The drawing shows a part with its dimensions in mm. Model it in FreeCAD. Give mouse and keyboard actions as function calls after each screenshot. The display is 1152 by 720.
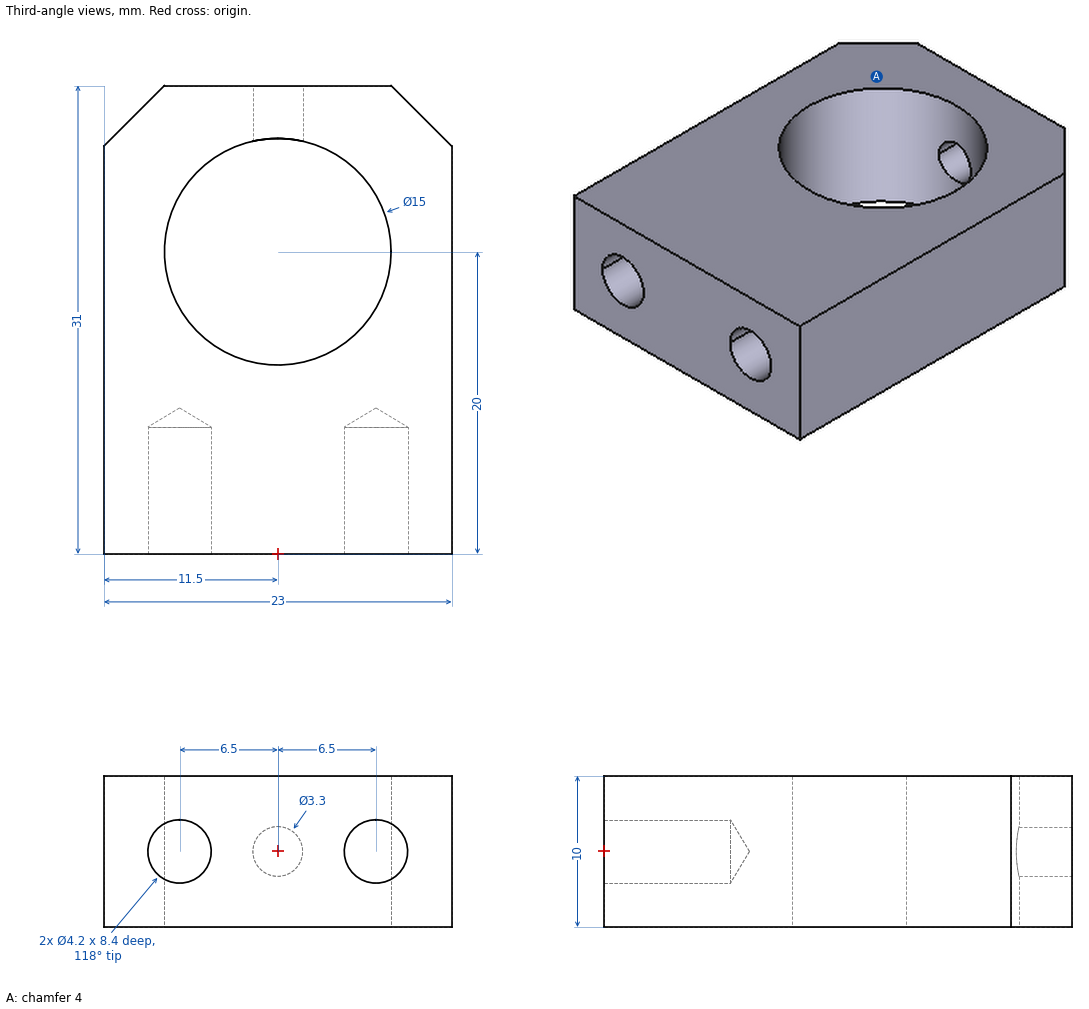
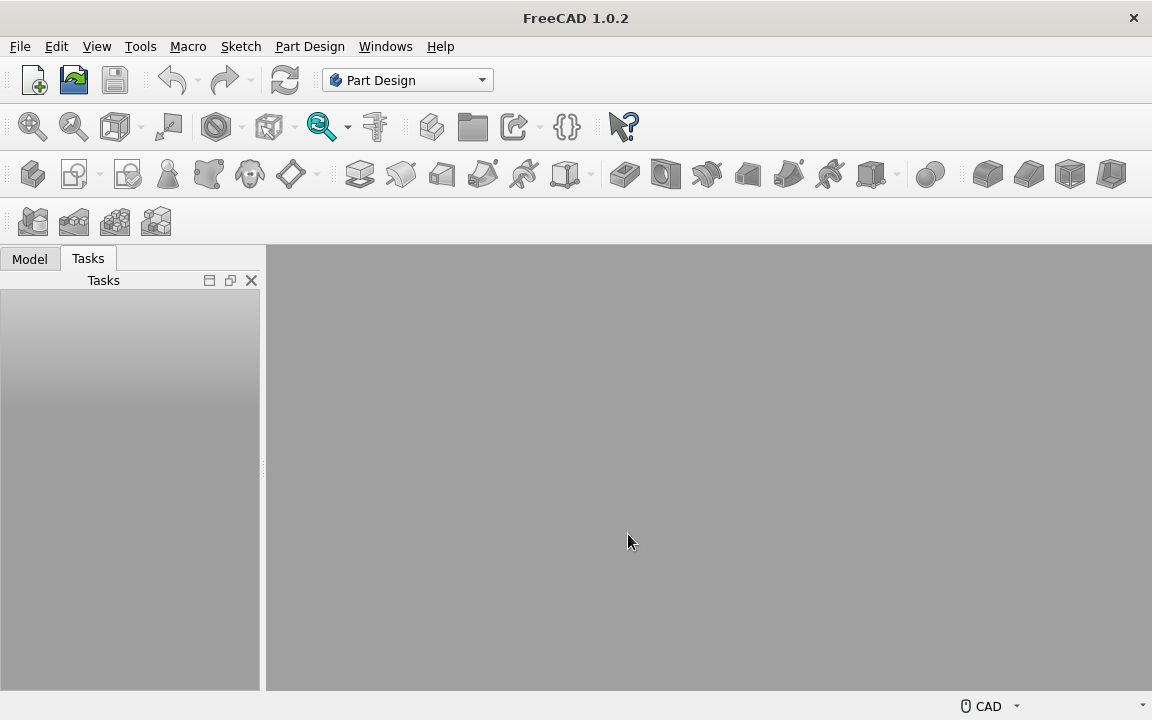
key(ctrl+n)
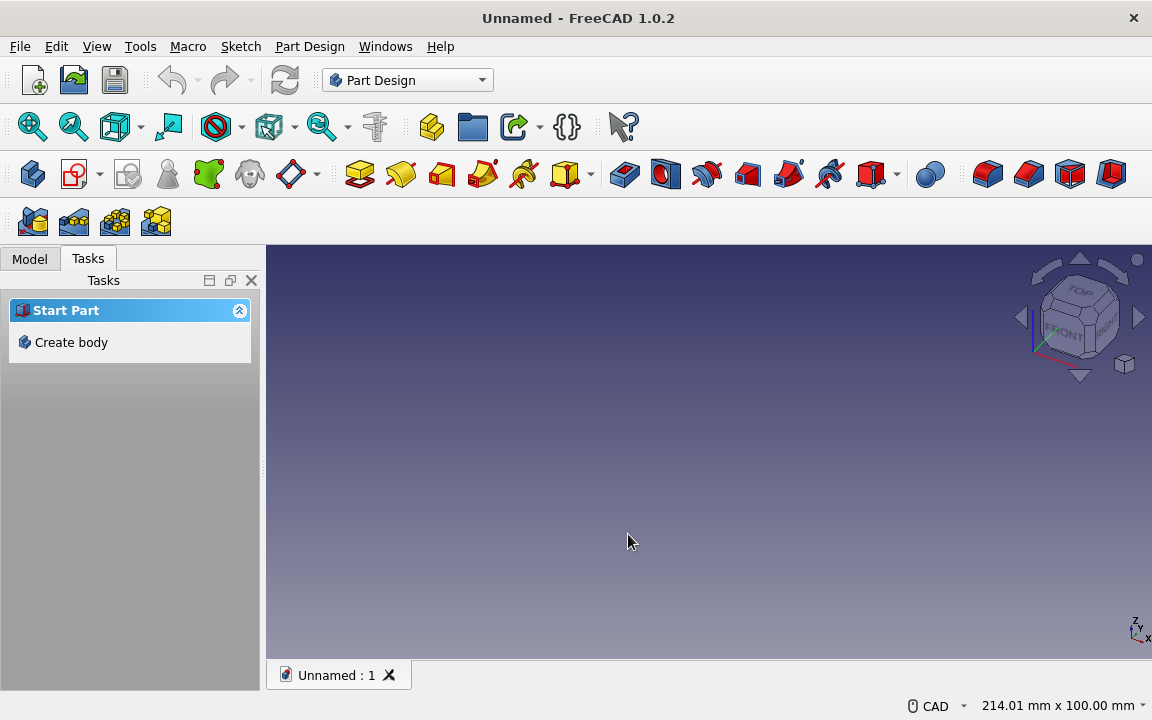
click(74, 174)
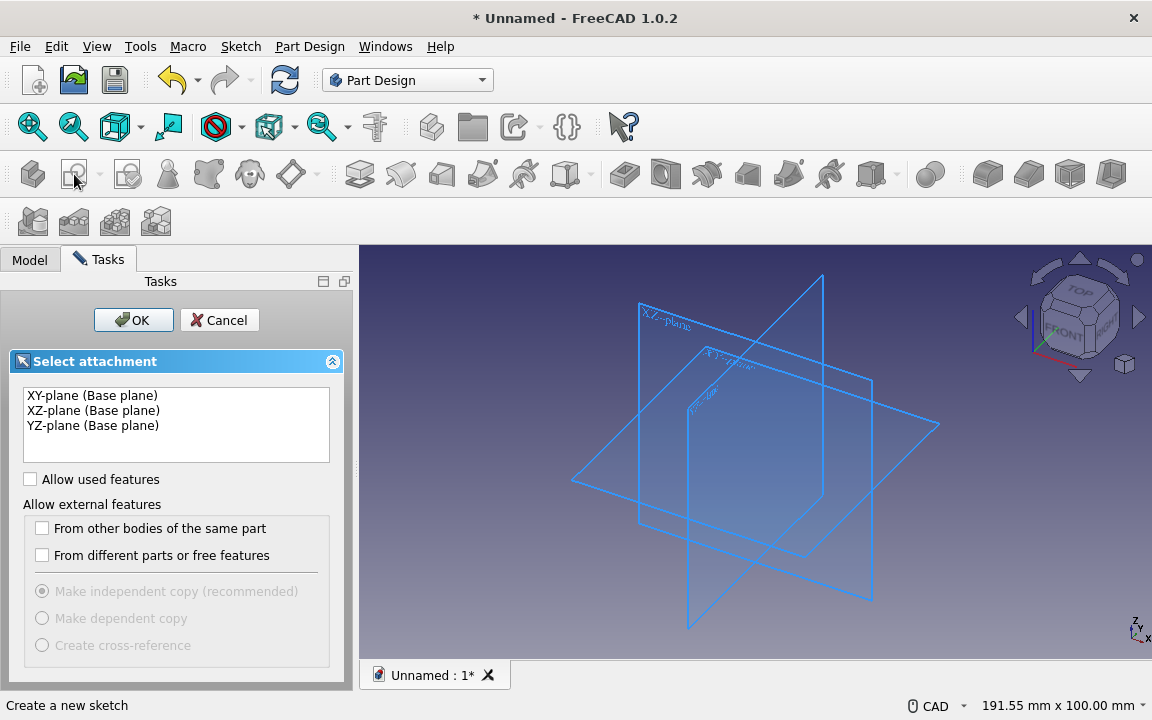
click(84, 396)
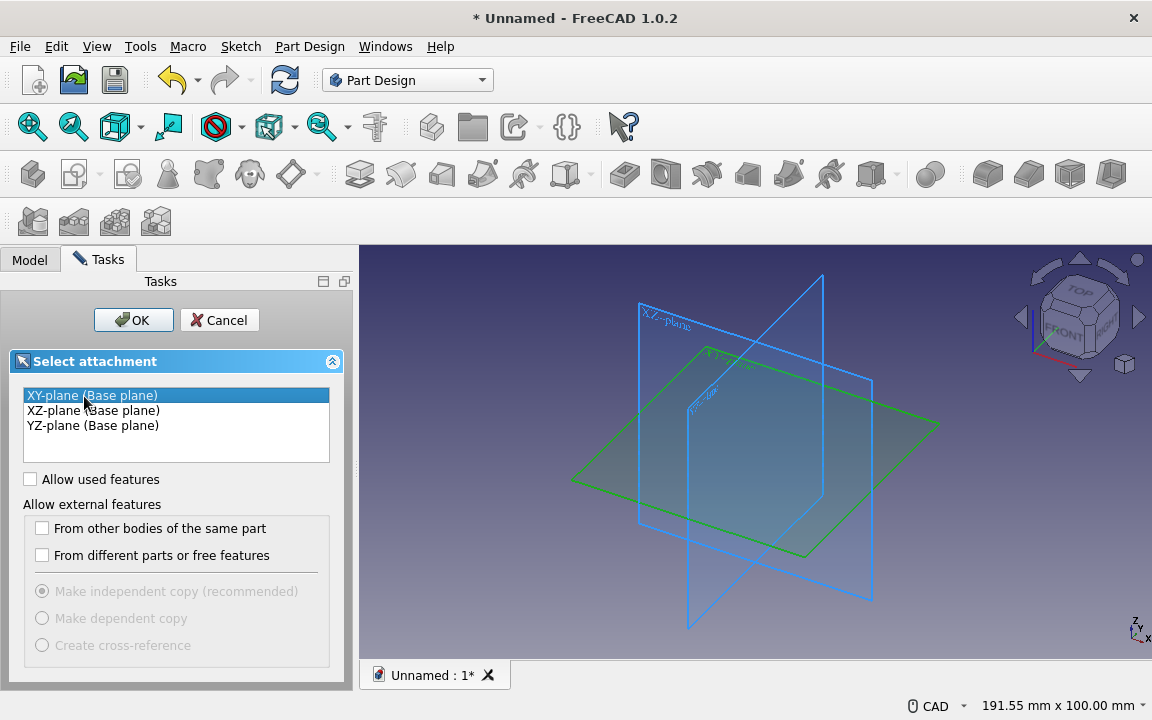
click(134, 320)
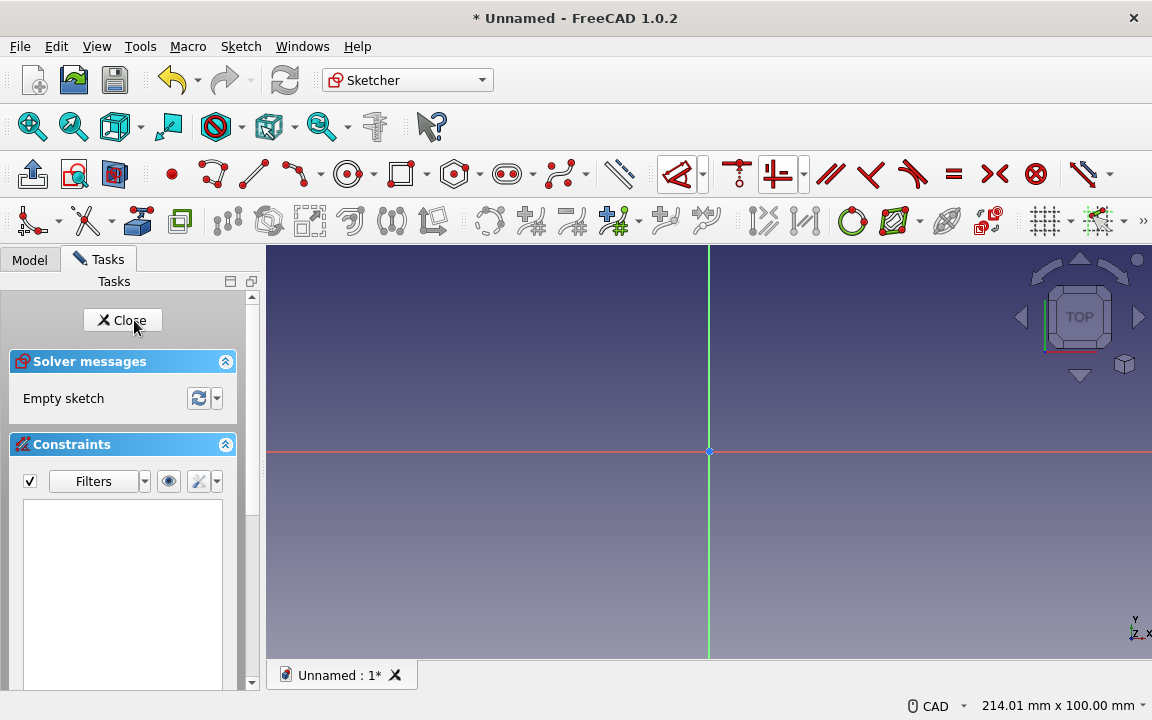
scroll(792, 310, up, 3)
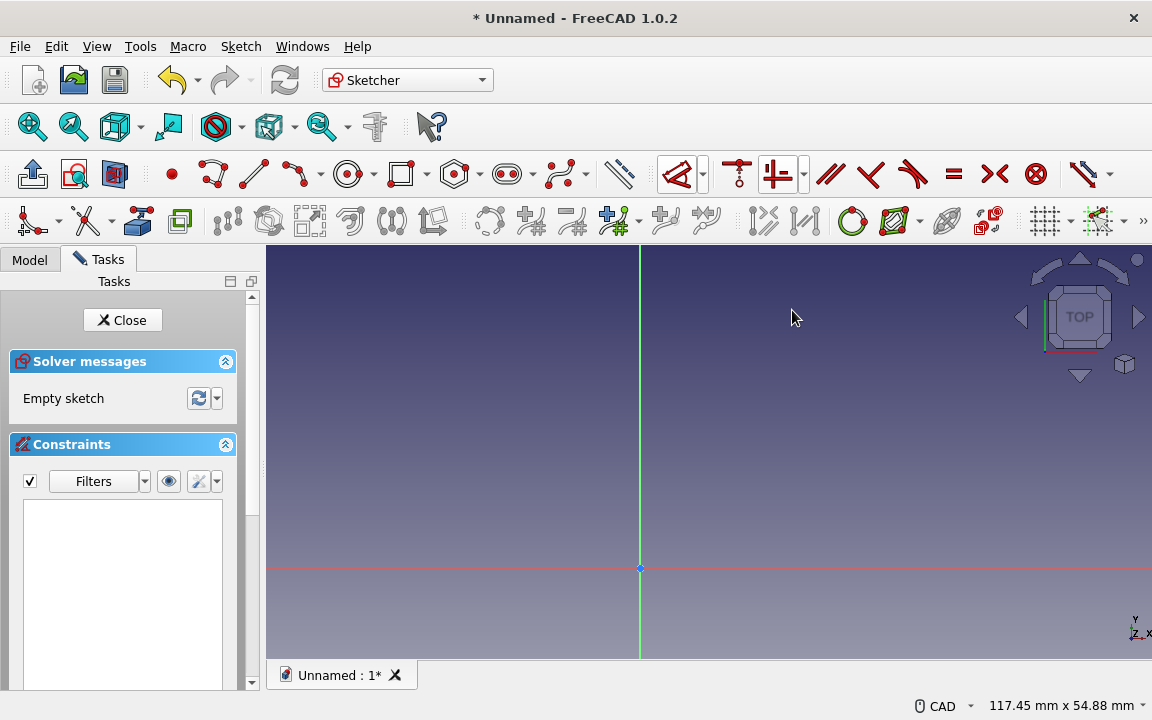
key(g)
key(r)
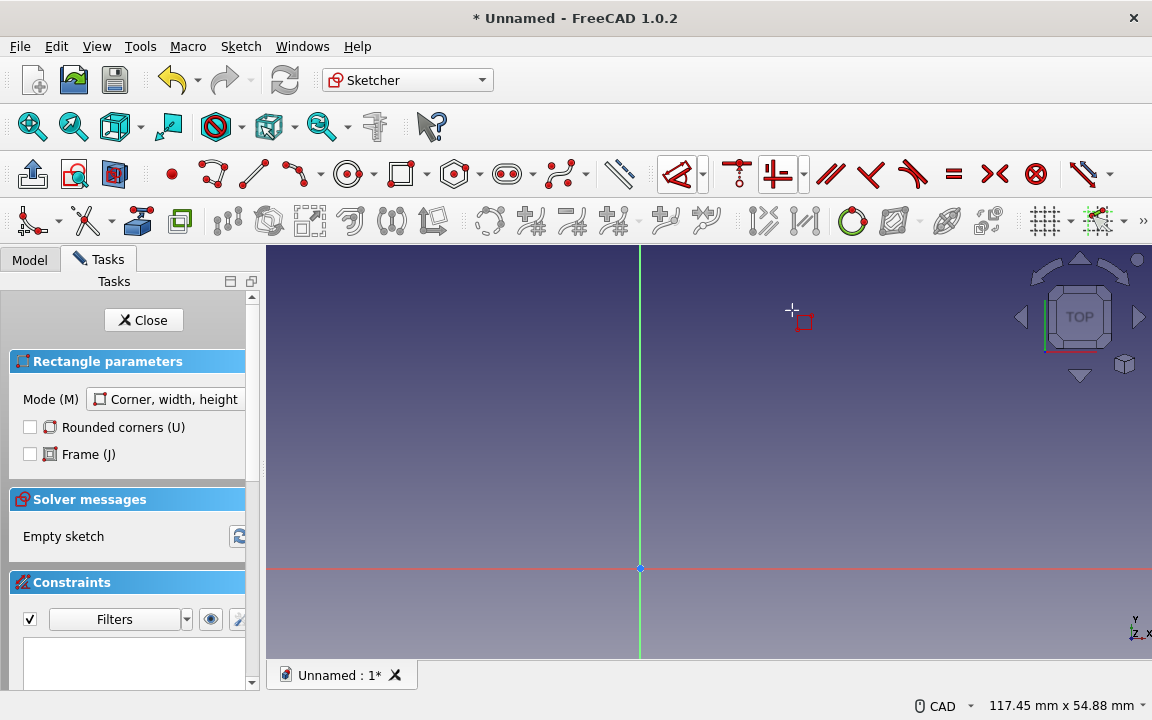
click(554, 335)
click(727, 569)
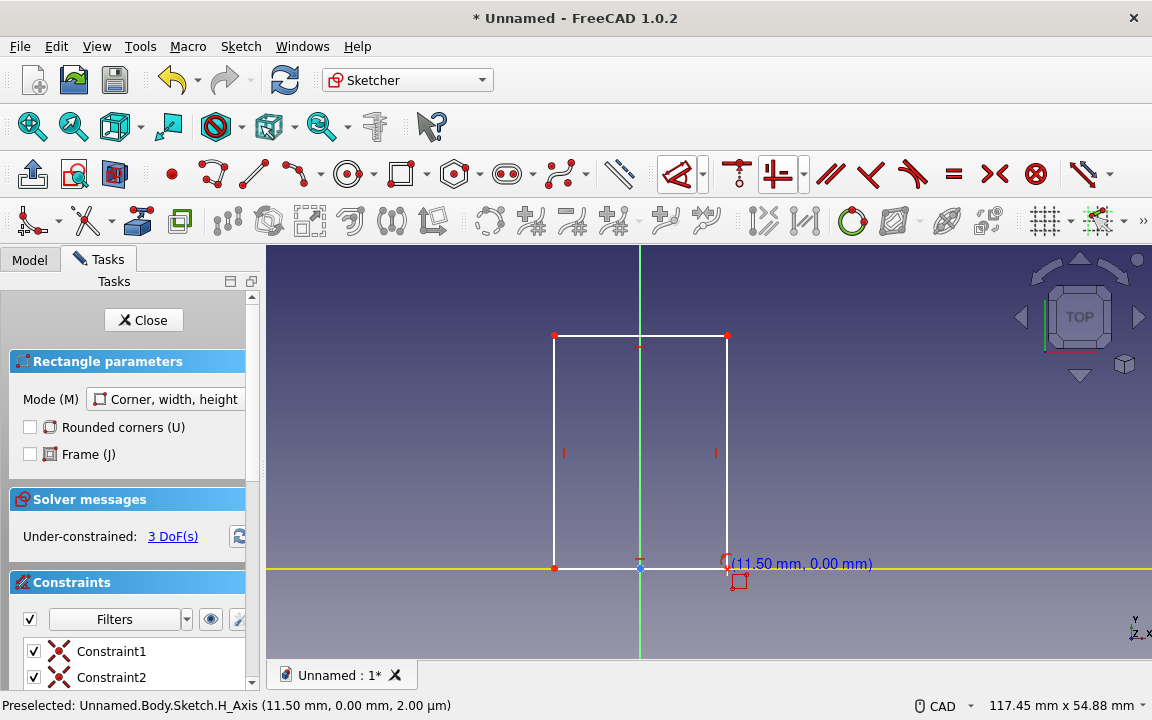
key(g)
key(c)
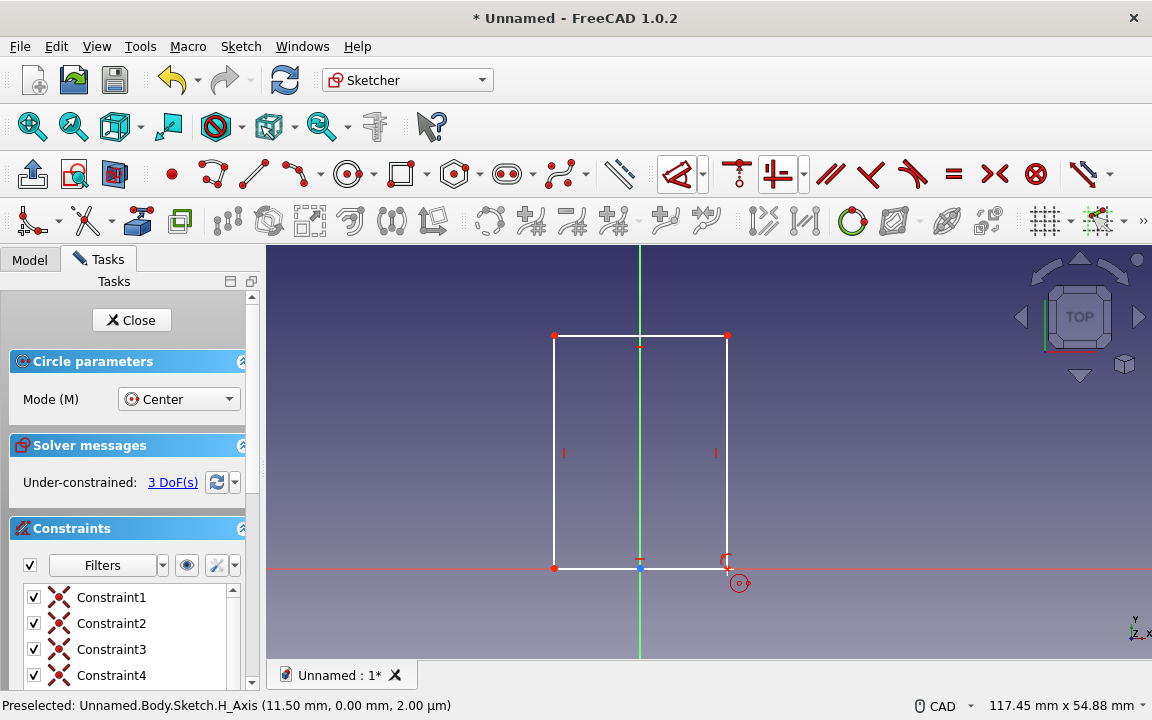
click(640, 418)
move(680, 378)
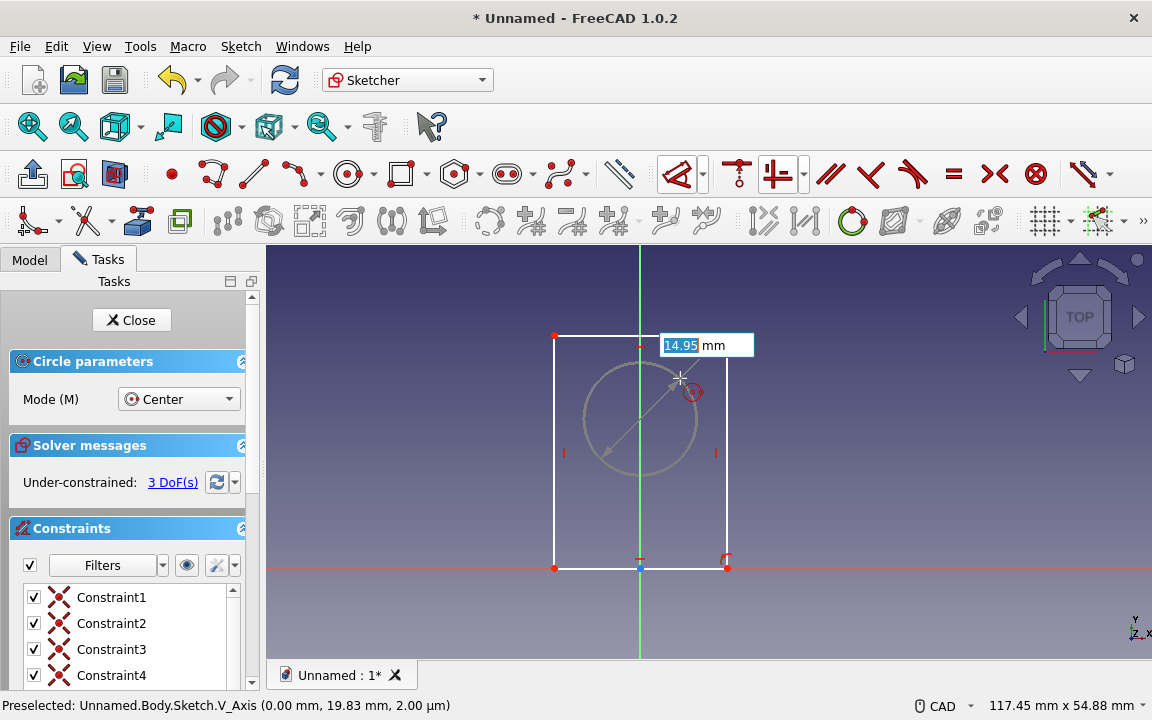
text(15)
key(Return)
key(Escape)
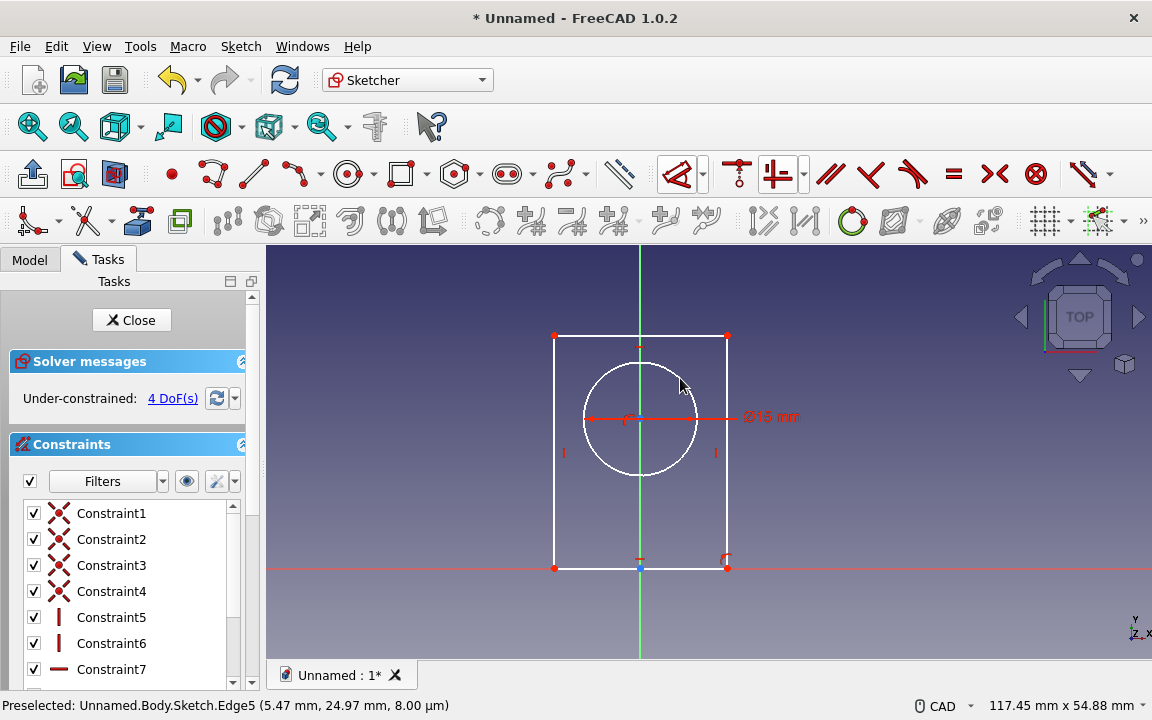
key(d)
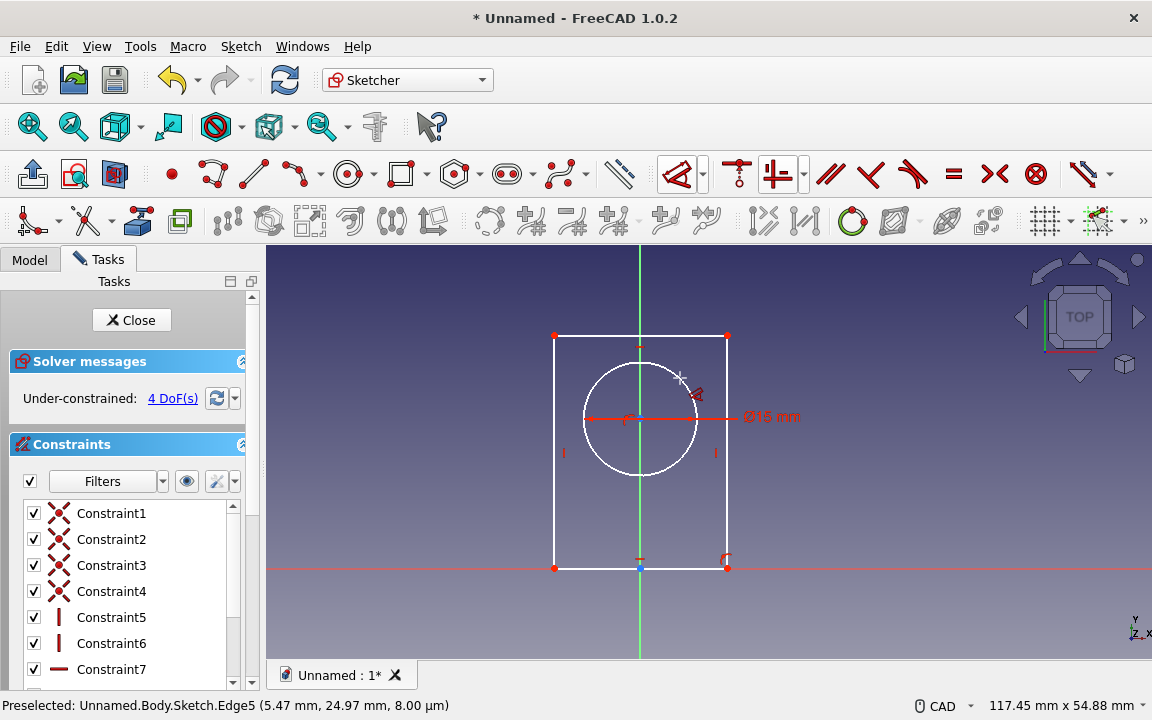
click(554, 406)
click(520, 452)